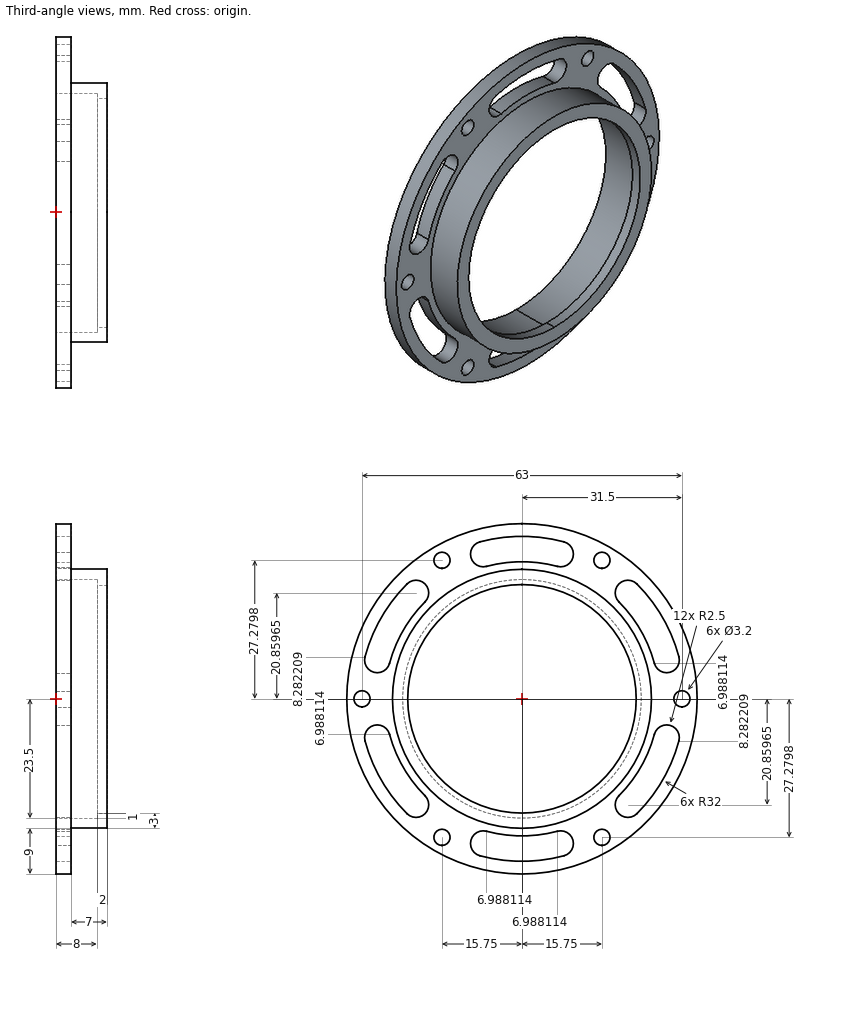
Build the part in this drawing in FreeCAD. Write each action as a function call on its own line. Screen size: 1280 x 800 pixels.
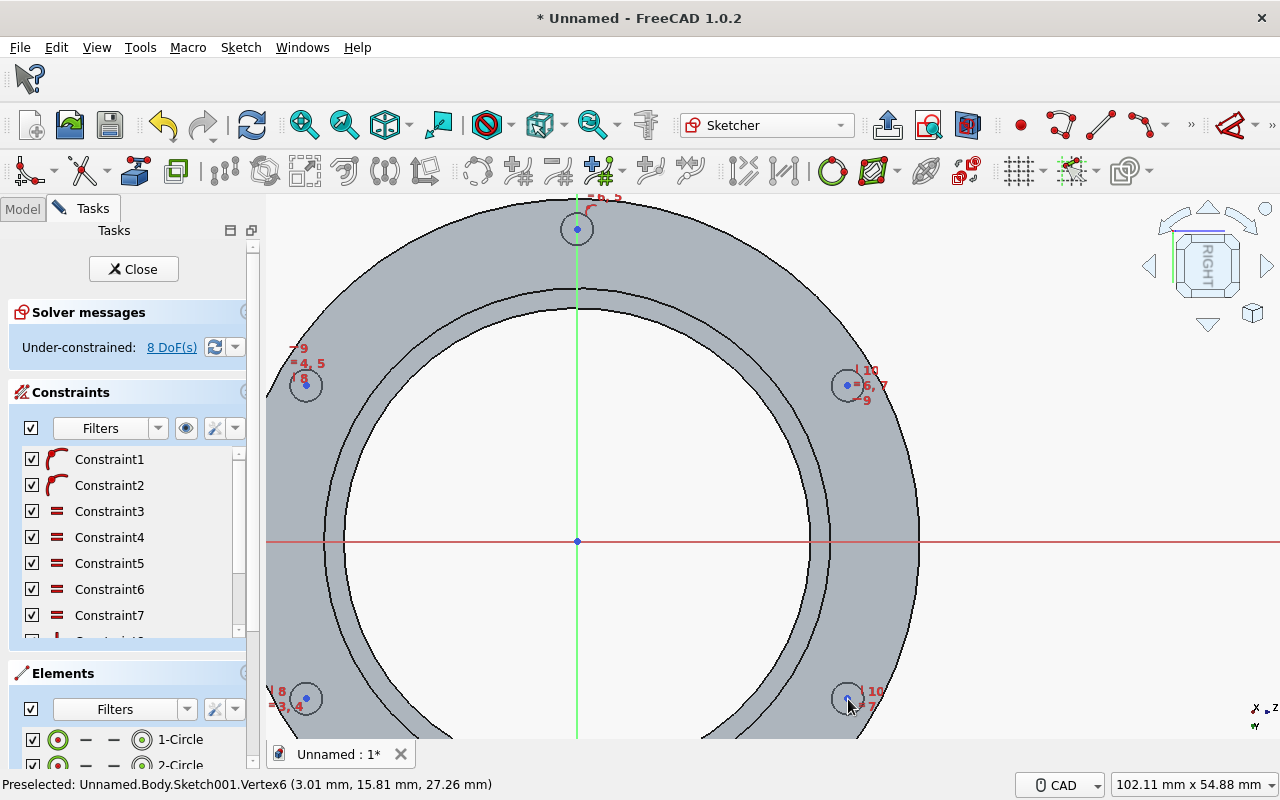
click(306, 699)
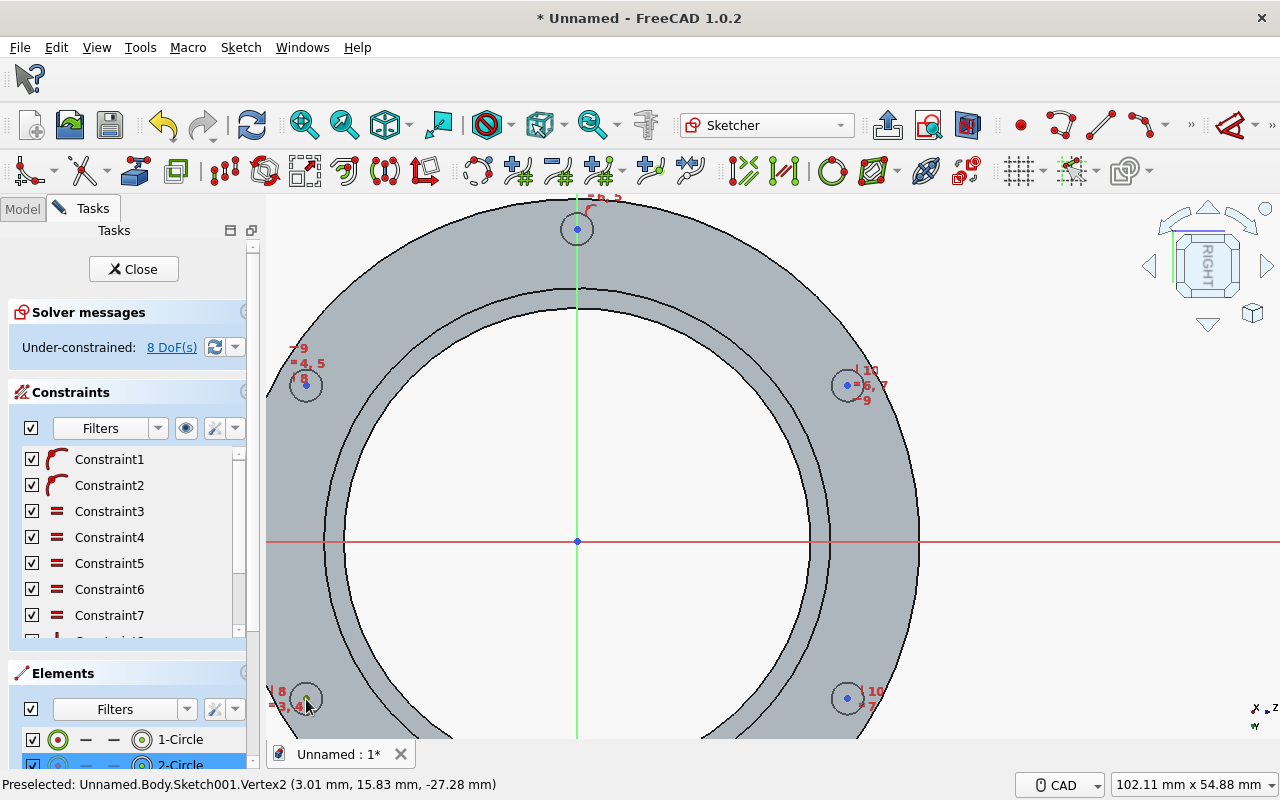
click(848, 699)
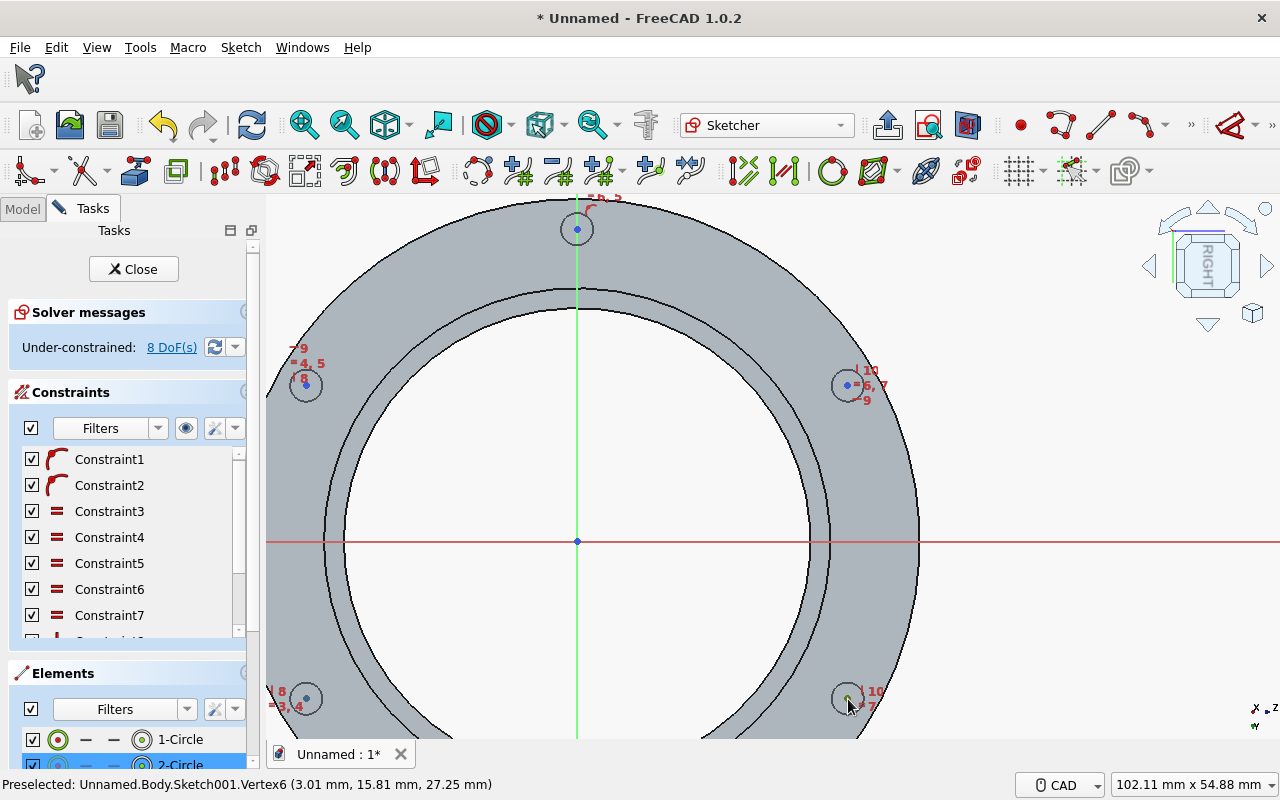
key(h)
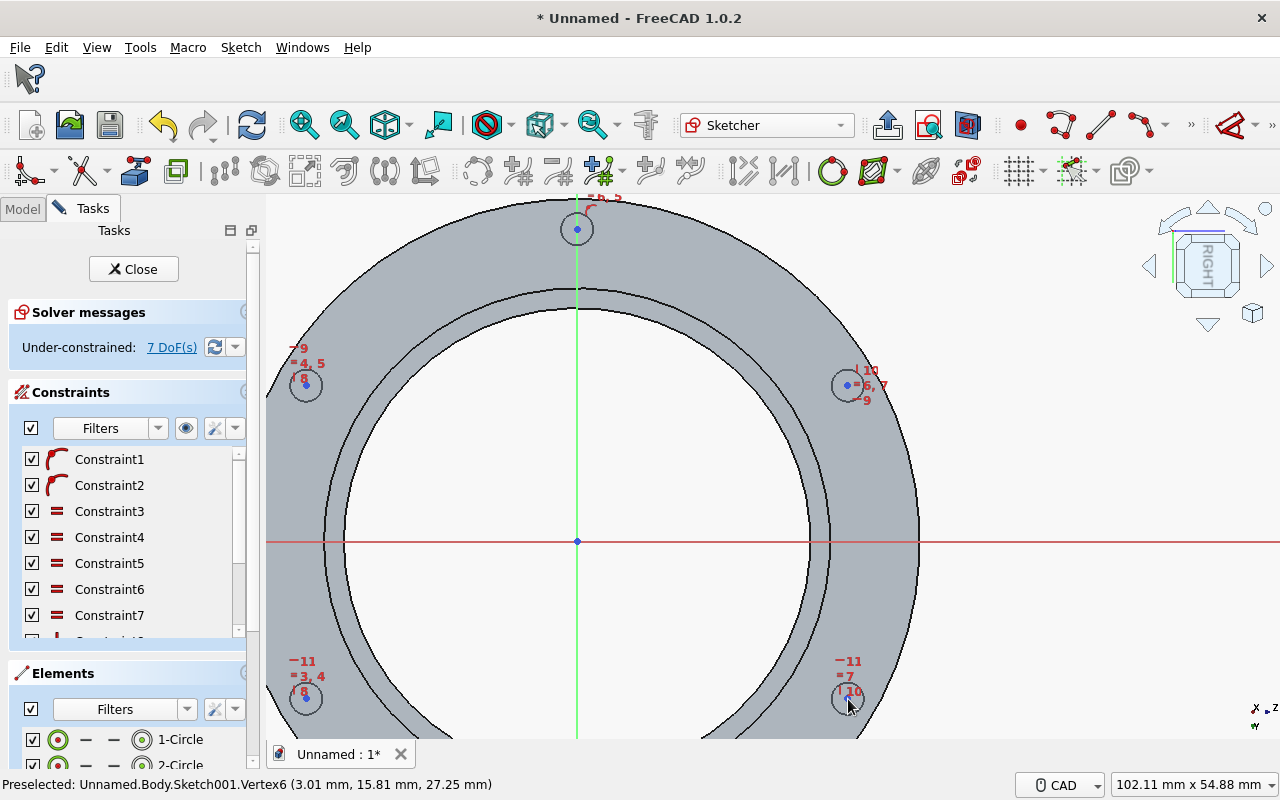
key(d)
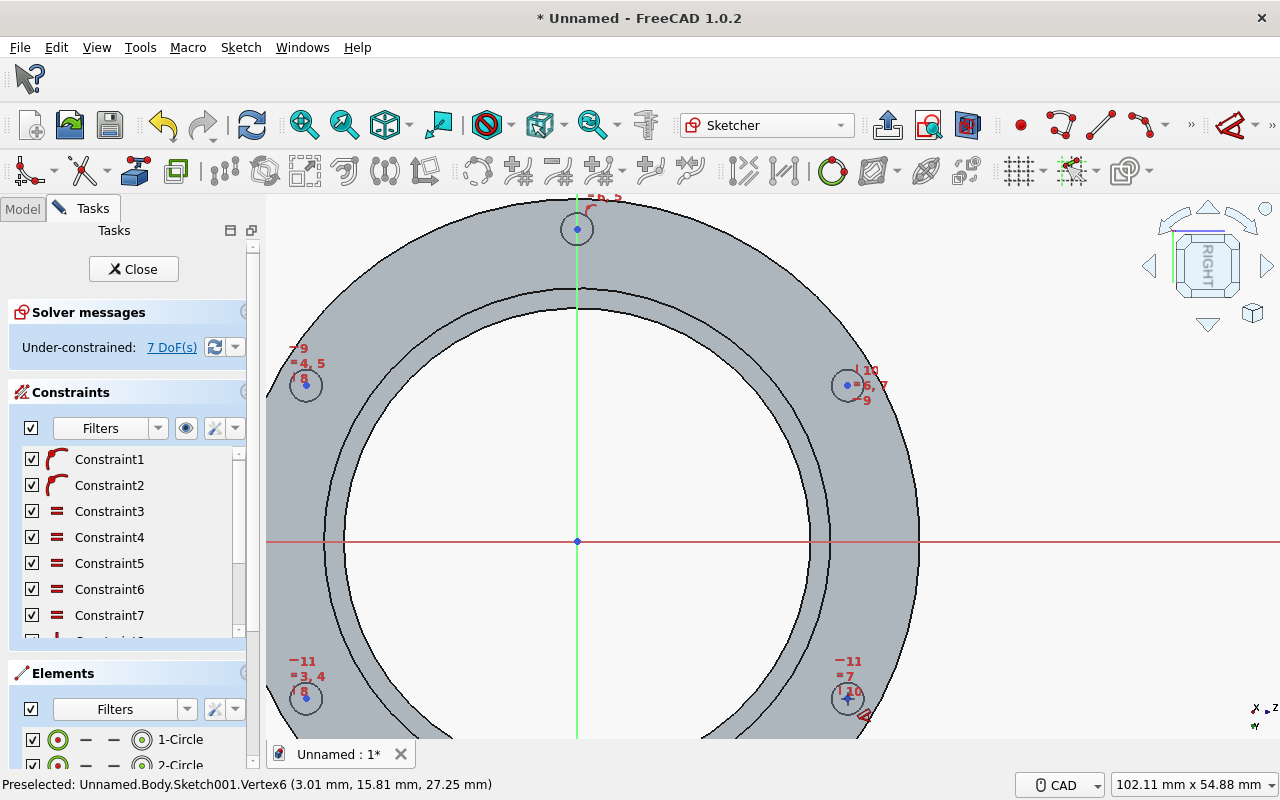
scroll(859, 375, down, 3)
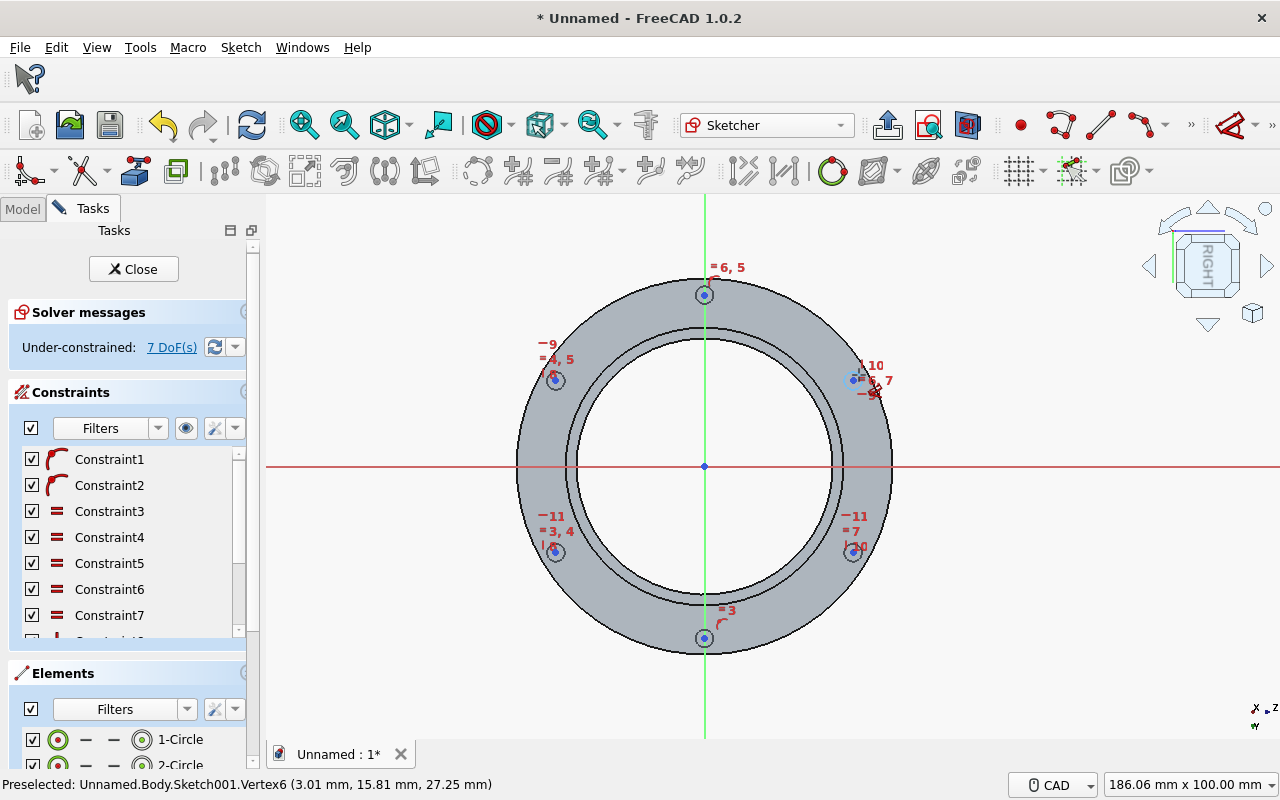
scroll(711, 632, up, 5)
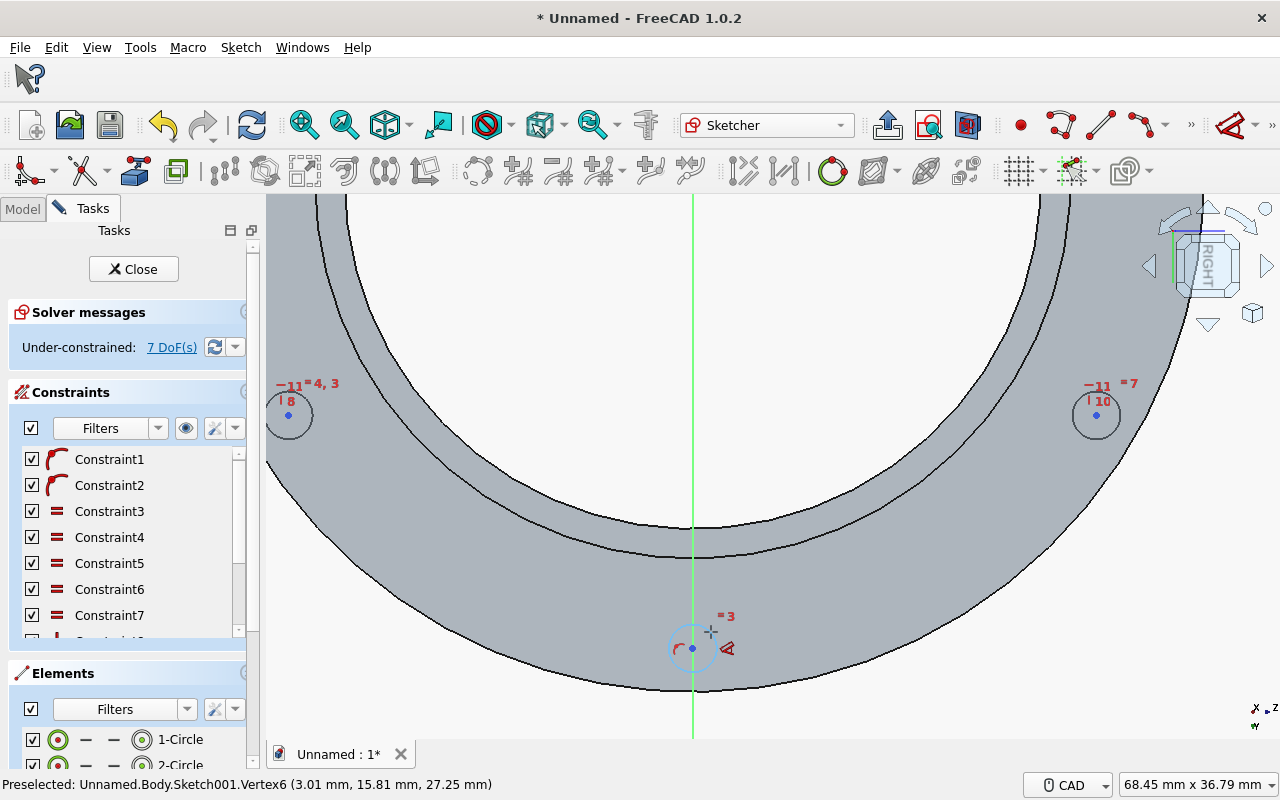
click(710, 631)
click(733, 608)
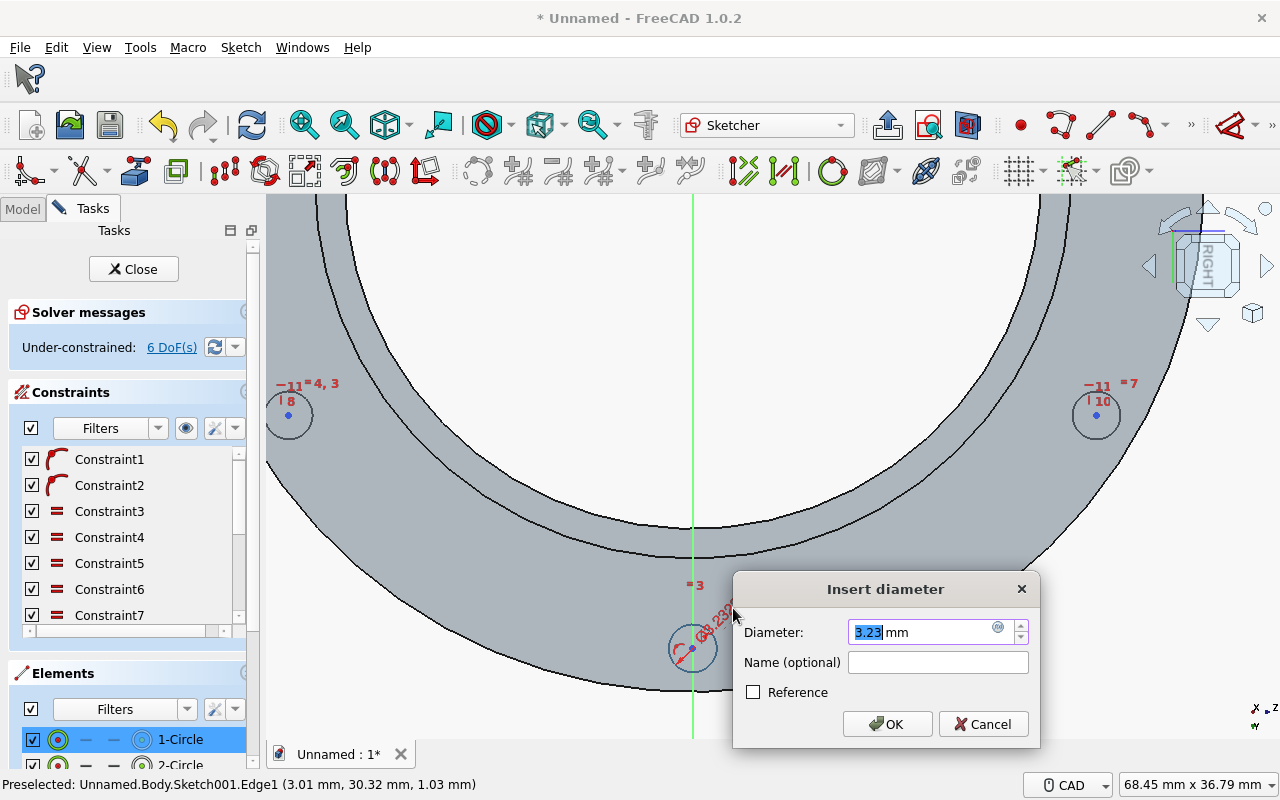
text(3.2)
key(Return)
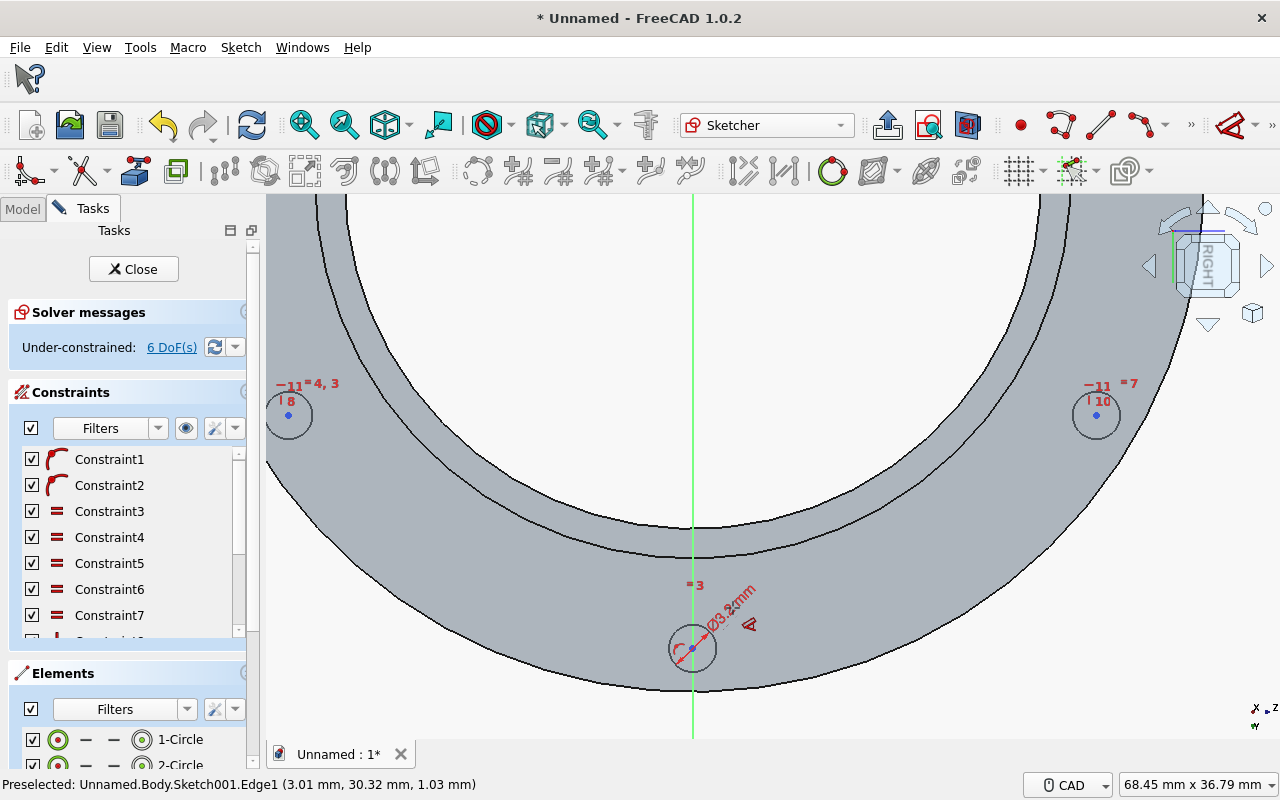
click(693, 648)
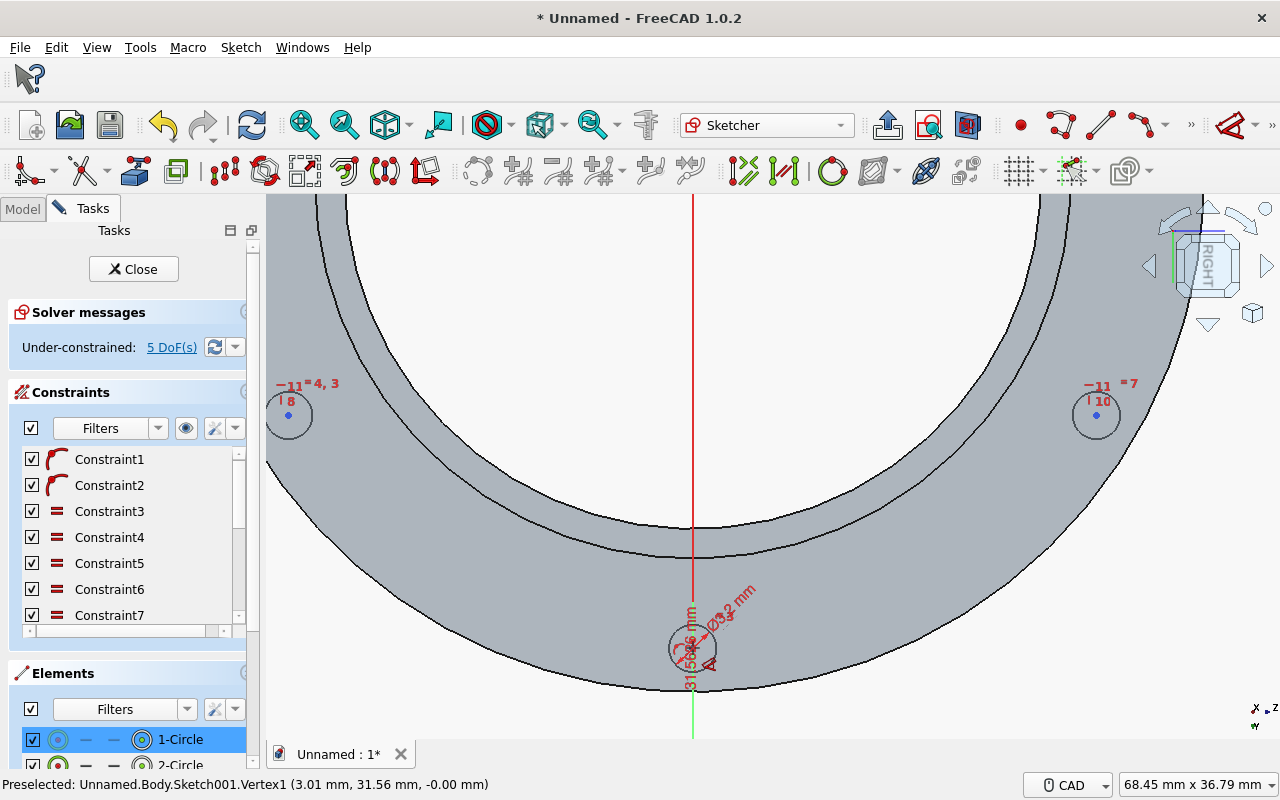
scroll(711, 633, down, 5)